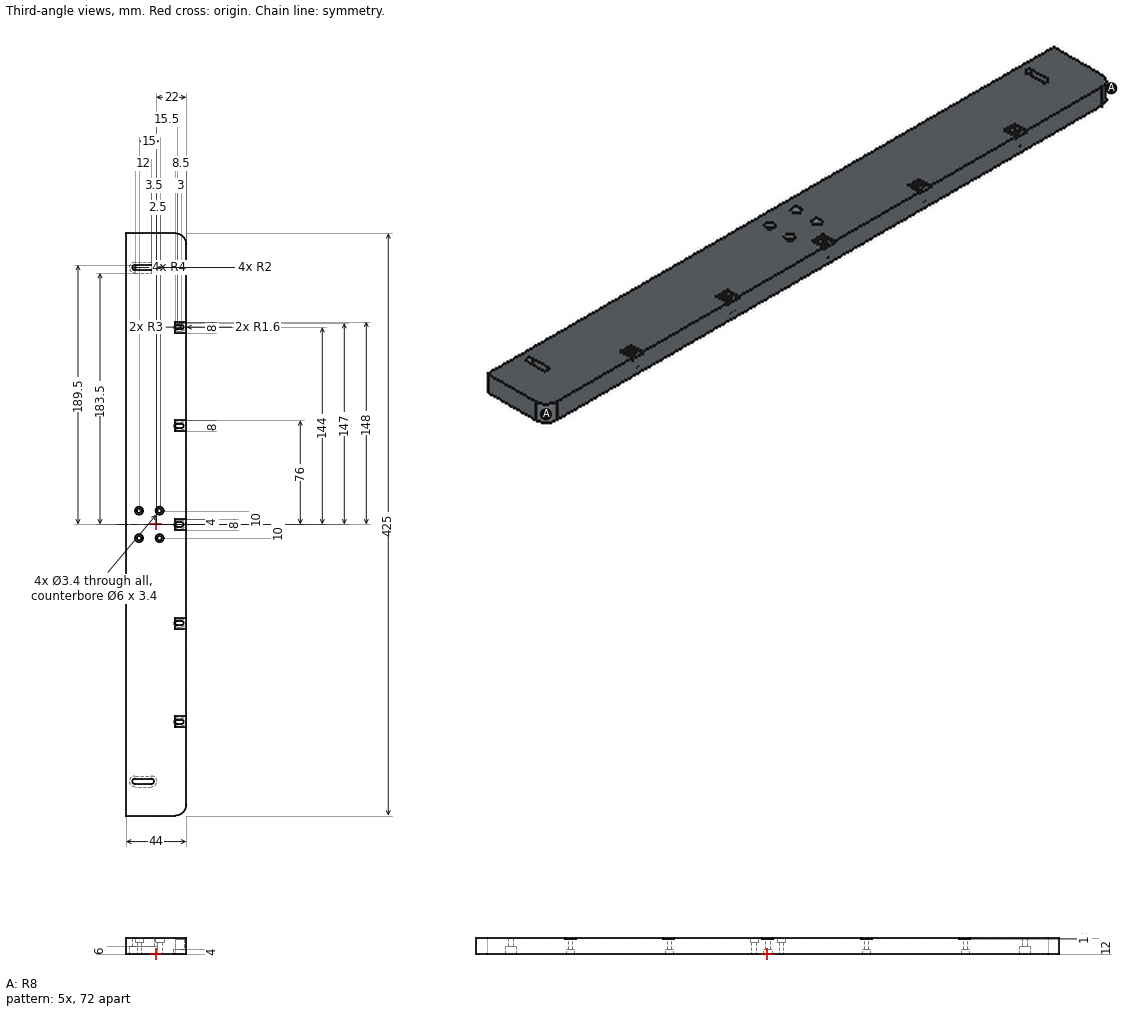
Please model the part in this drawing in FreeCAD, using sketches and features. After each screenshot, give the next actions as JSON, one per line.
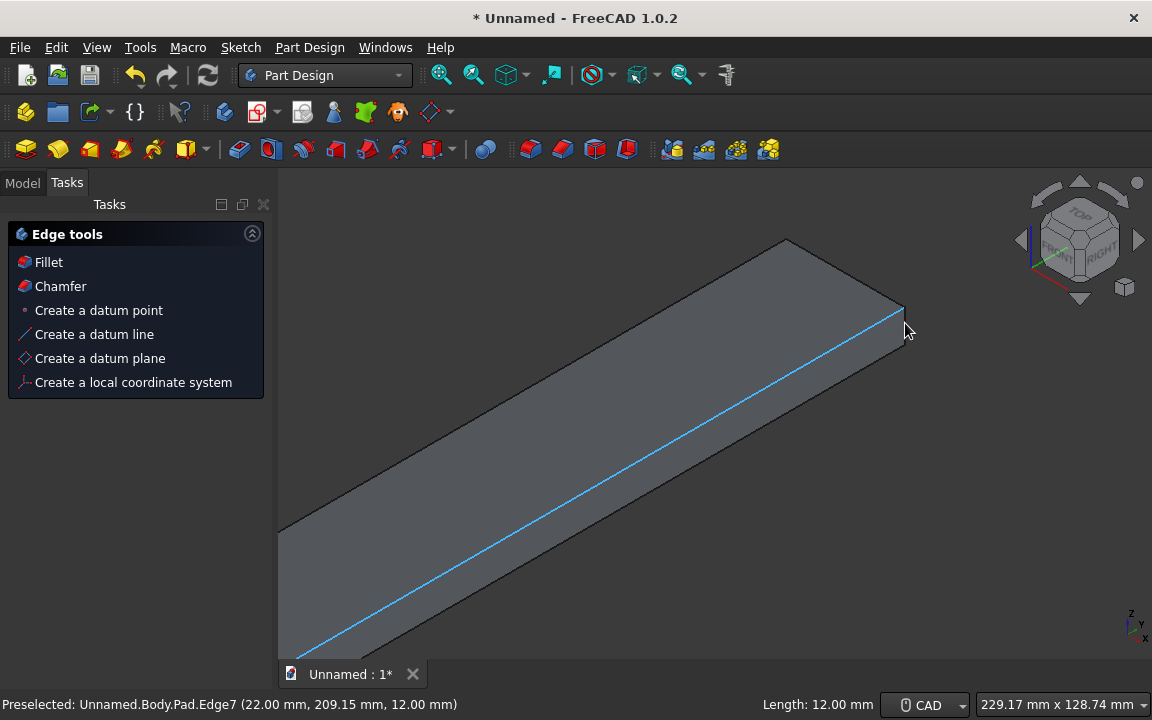
{"action": "key", "text": "v f"}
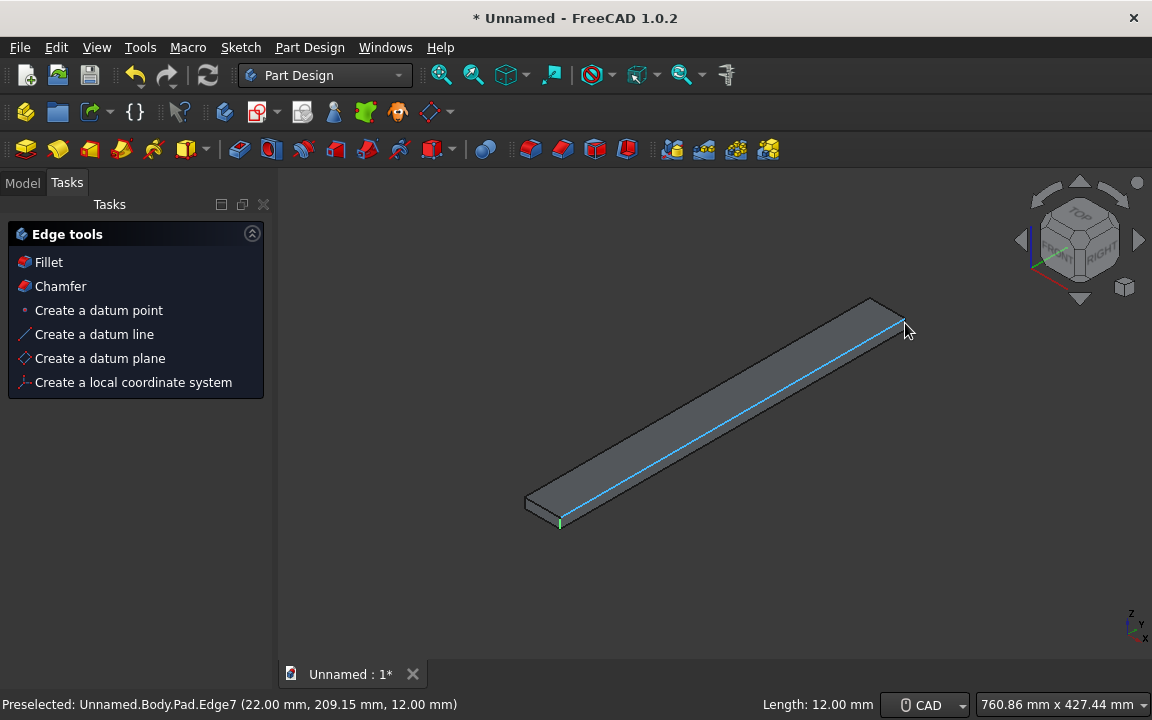
{"action": "key", "text": "2"}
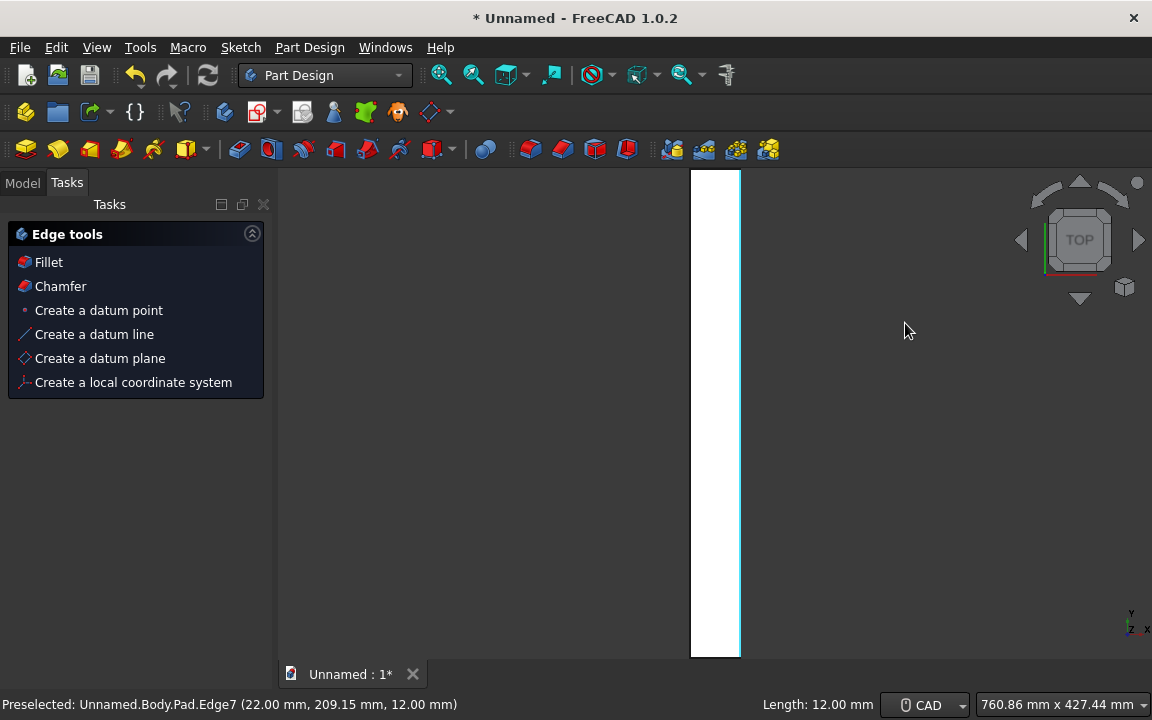
{"action": "key", "text": "1"}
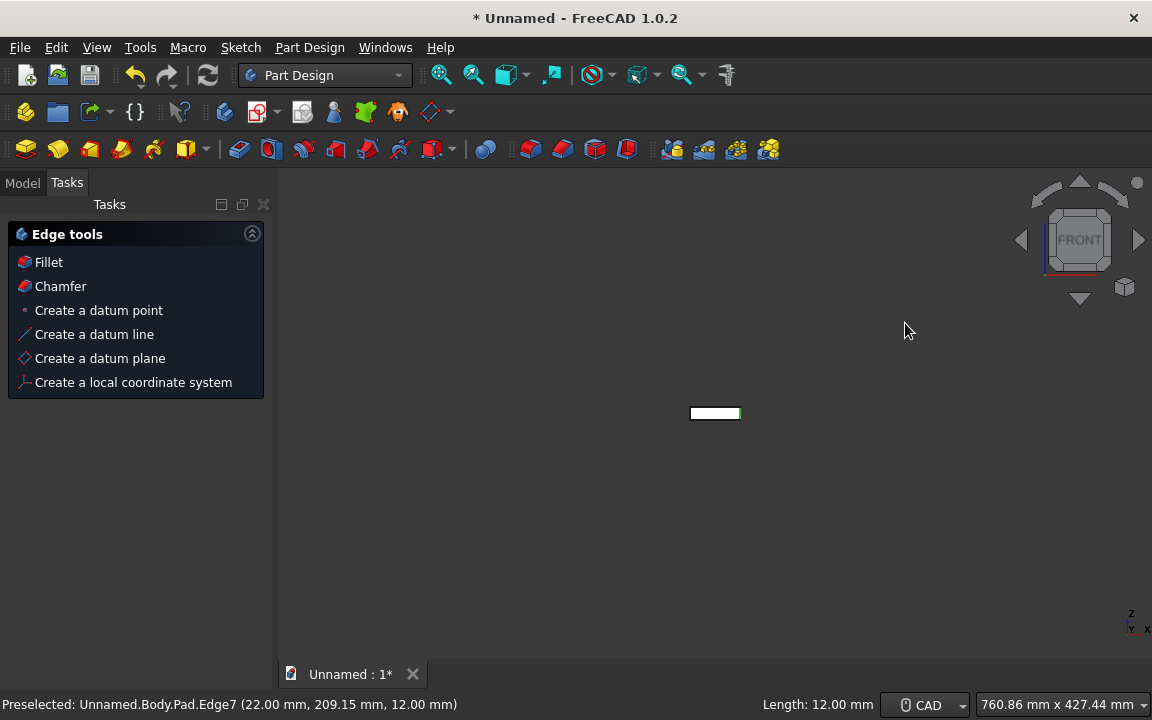
{"action": "key", "text": "v f"}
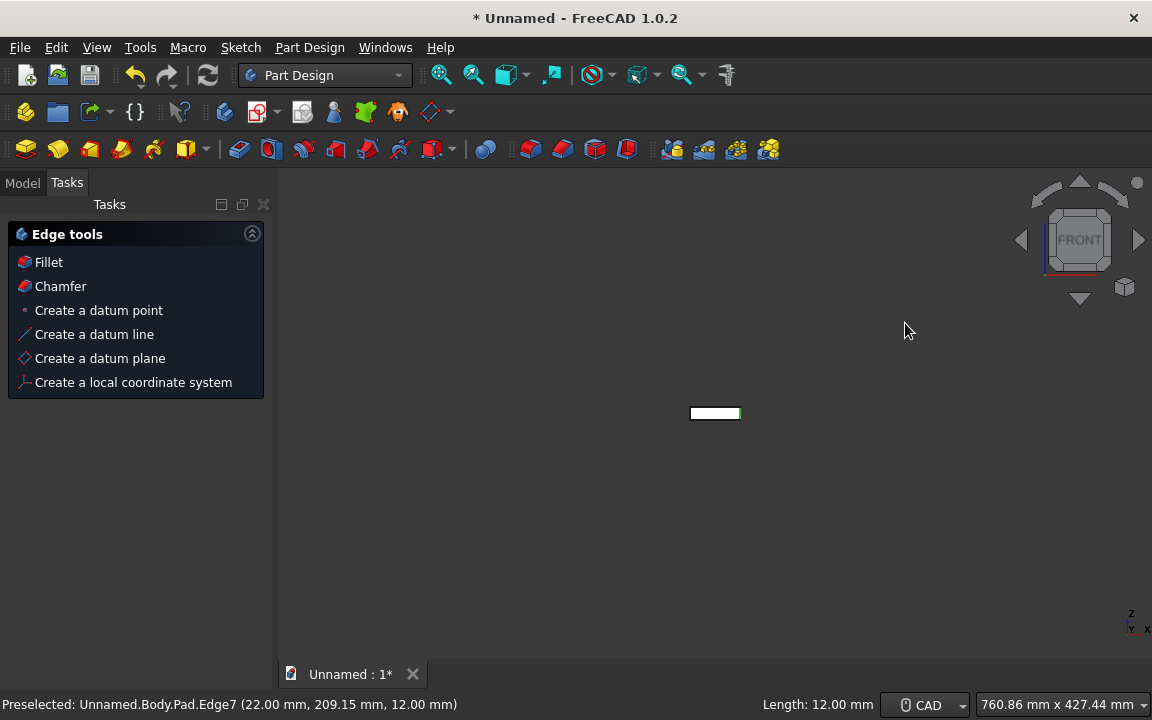
{"action": "scroll", "coordinate": [740, 413], "scroll_direction": "up", "scroll_amount": 6}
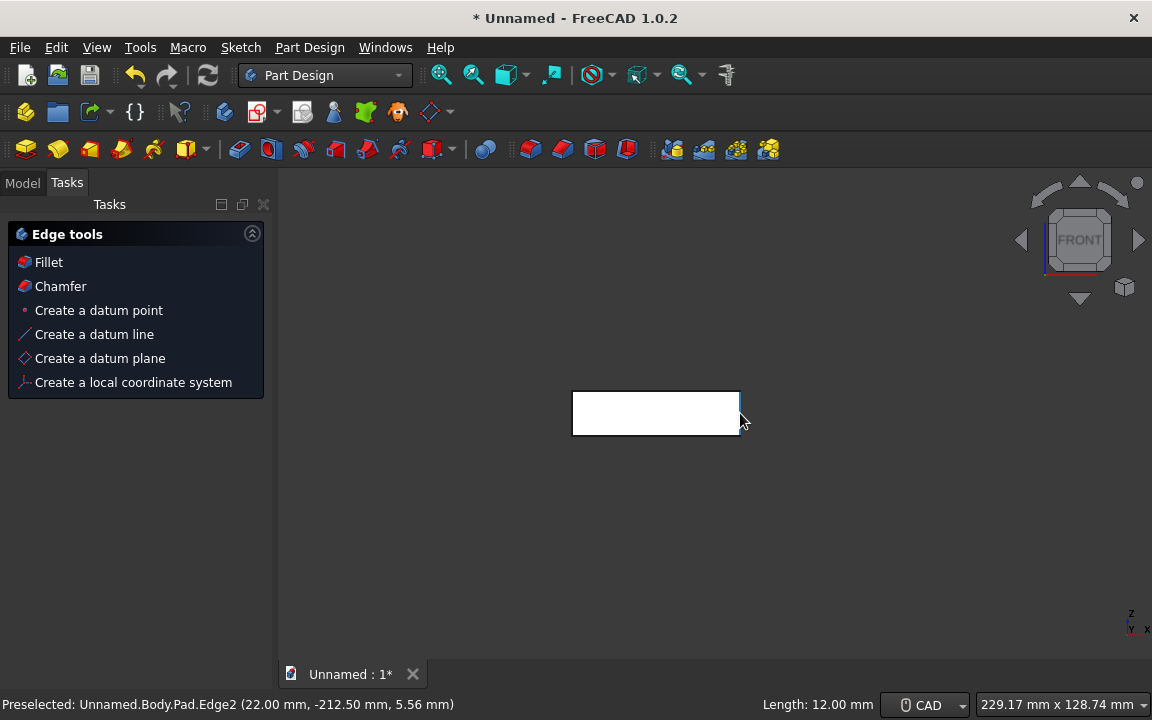
{"action": "key", "text": "v f"}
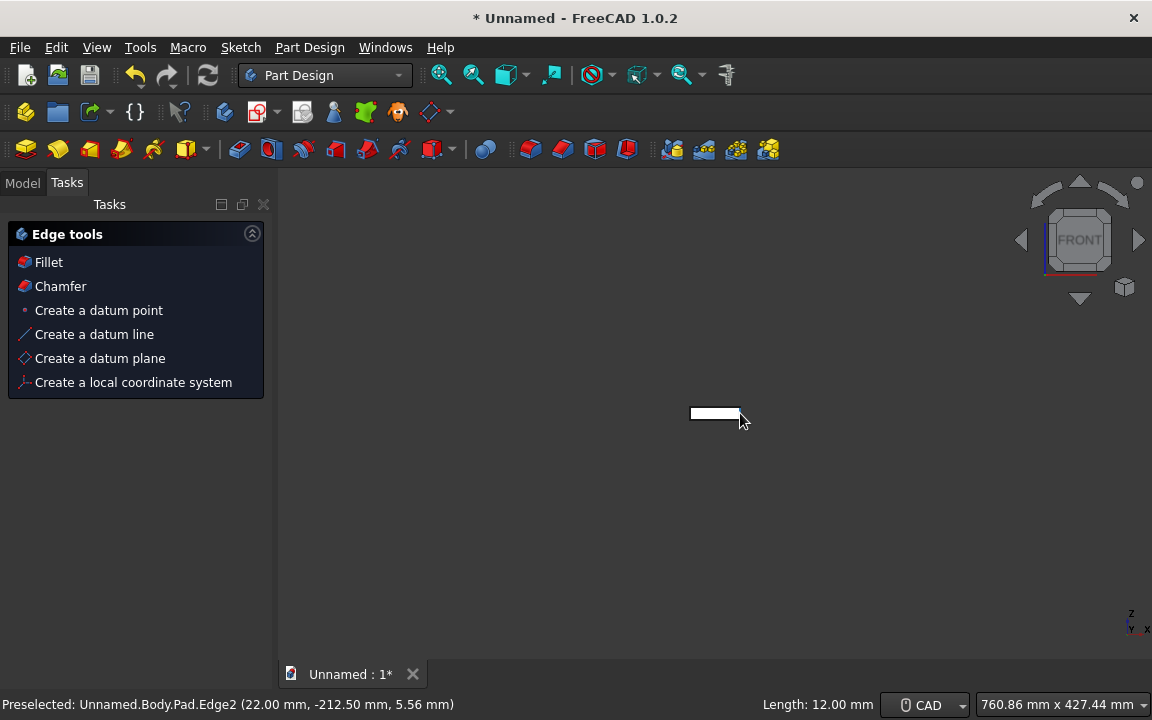
{"action": "key", "text": "3"}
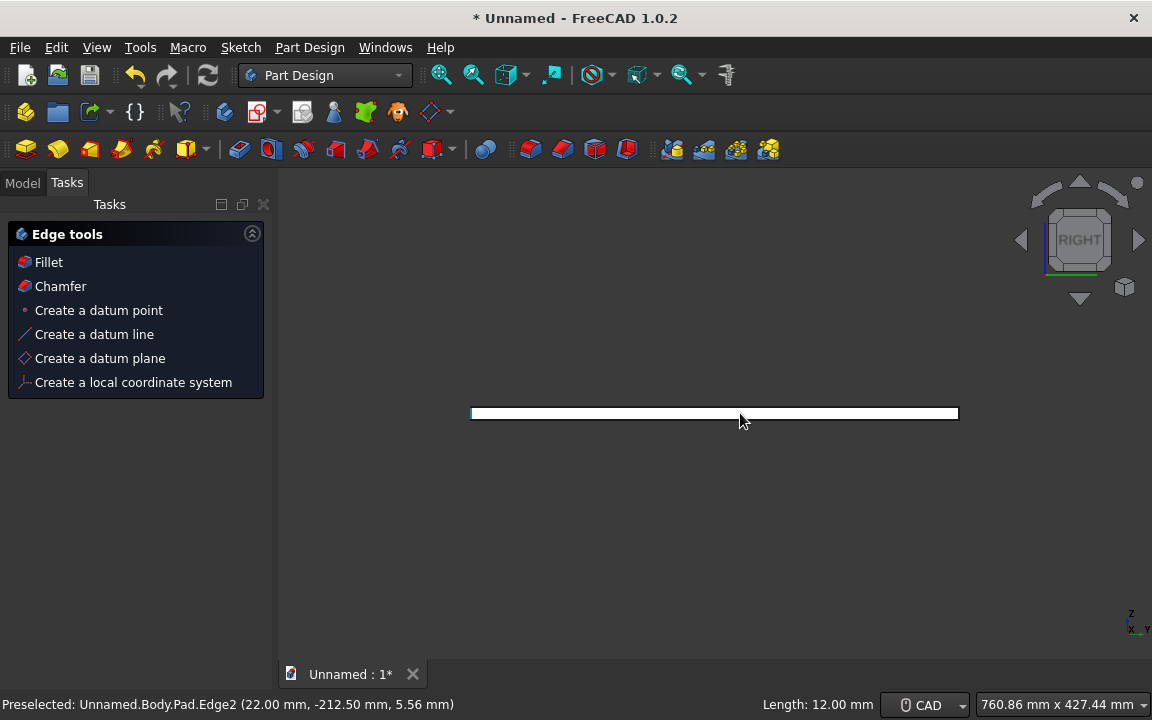
{"action": "left_click", "coordinate": [959, 412], "text": "ctrl"}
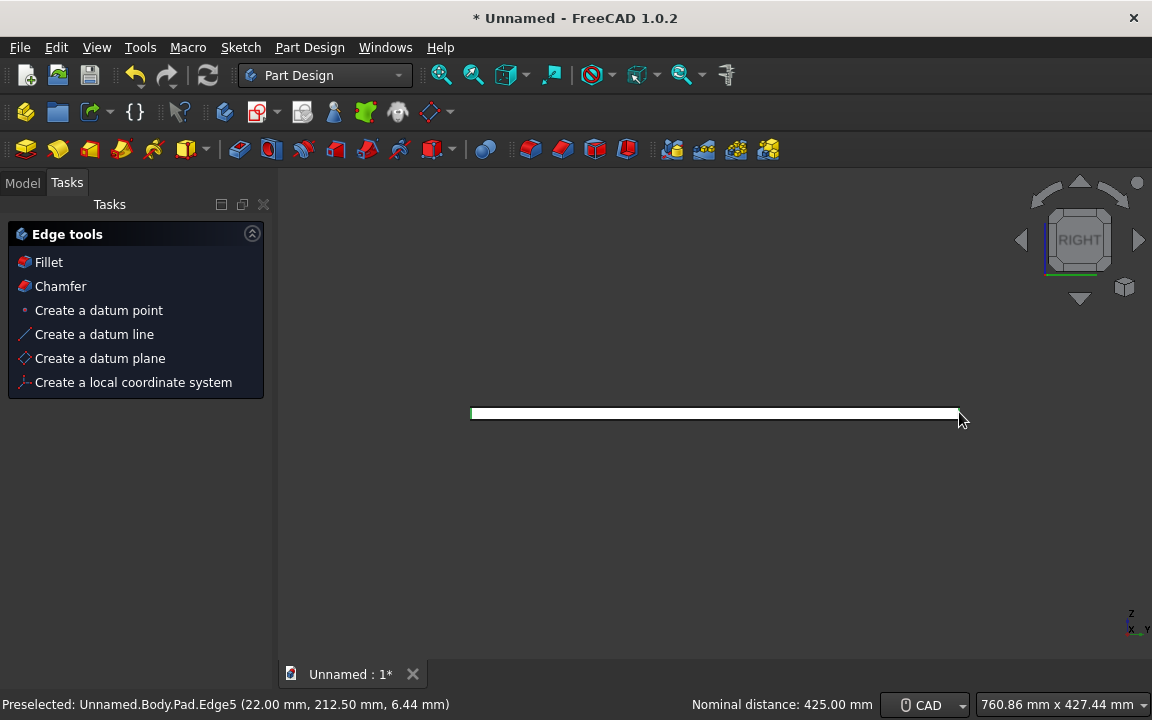
{"action": "left_click", "coordinate": [532, 150]}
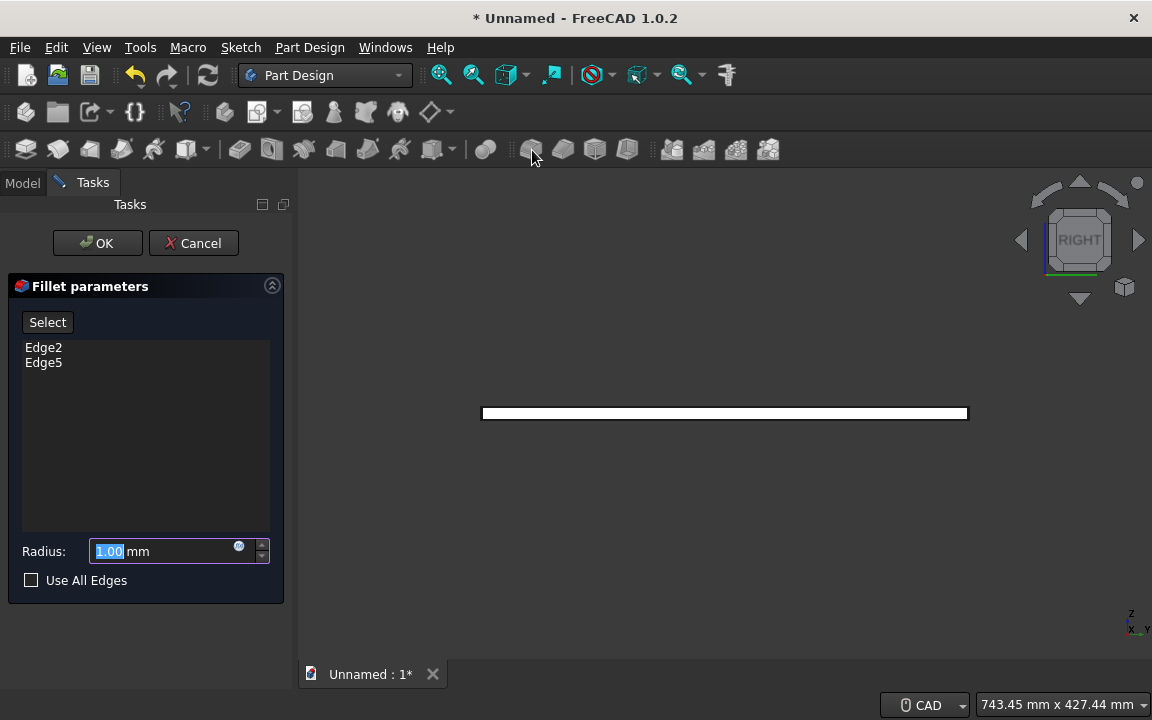
{"action": "type", "text": "8"}
{"action": "key", "text": "Tab"}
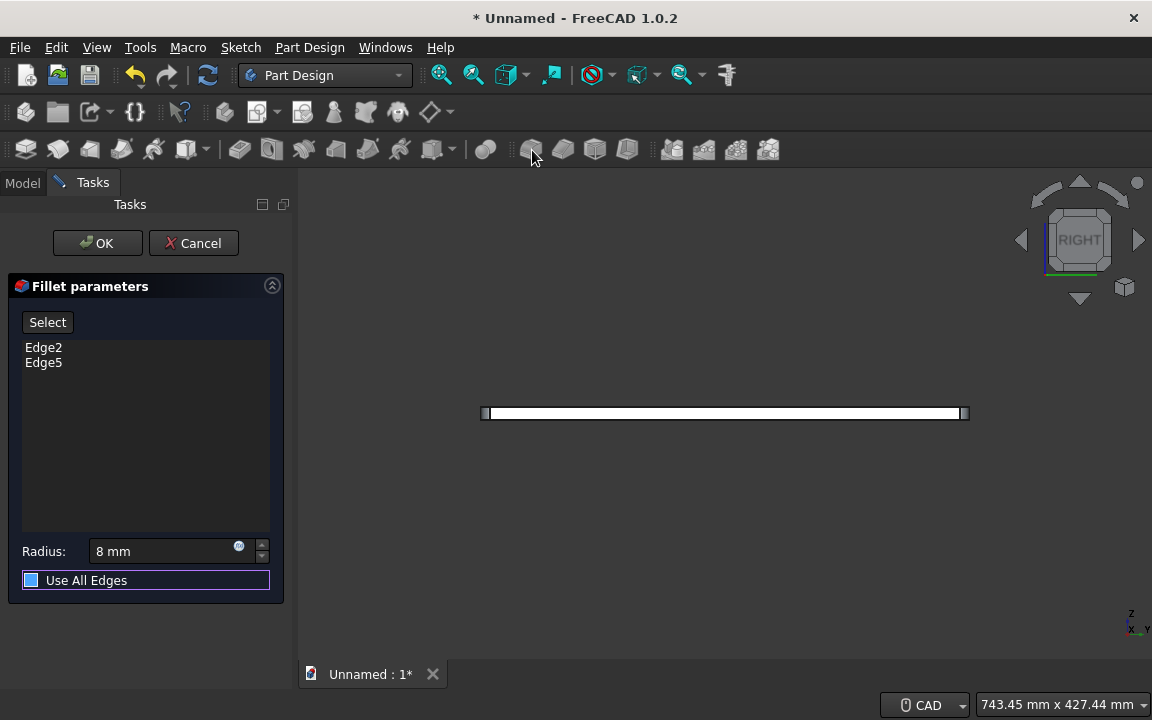
{"action": "left_click", "coordinate": [98, 243]}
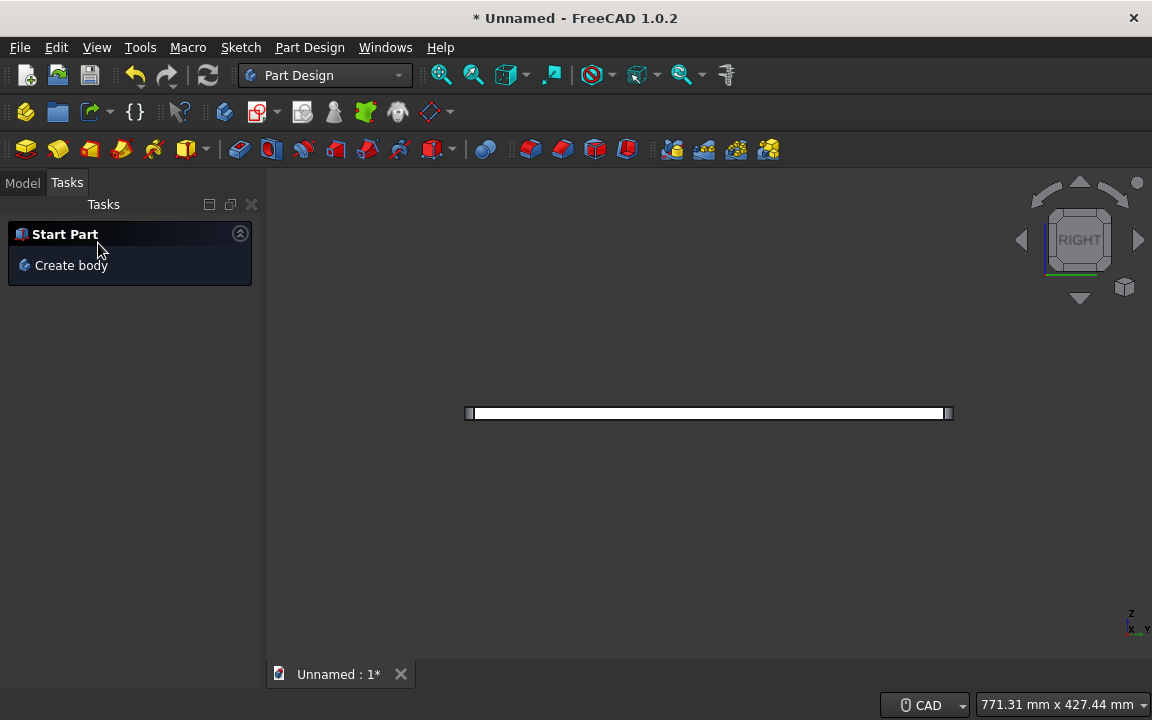
{"action": "key", "text": "5"}